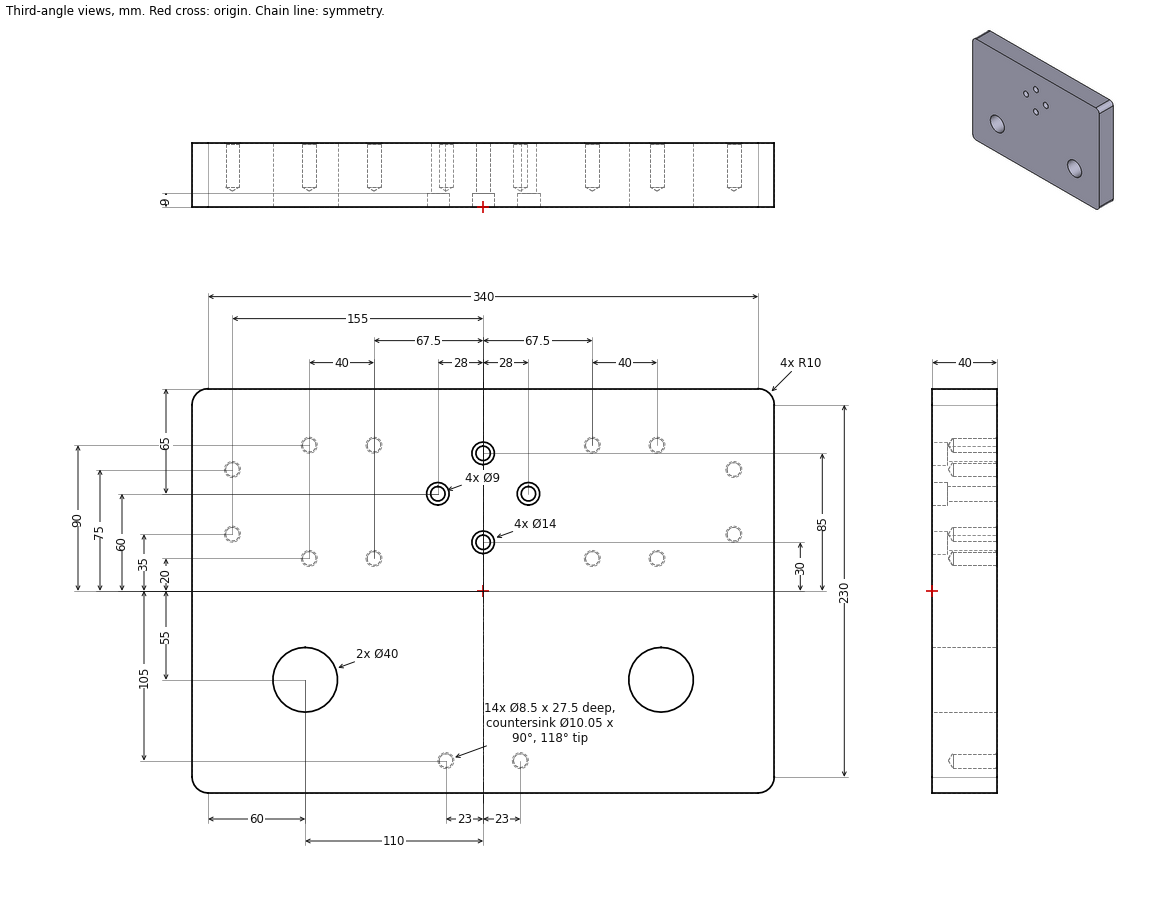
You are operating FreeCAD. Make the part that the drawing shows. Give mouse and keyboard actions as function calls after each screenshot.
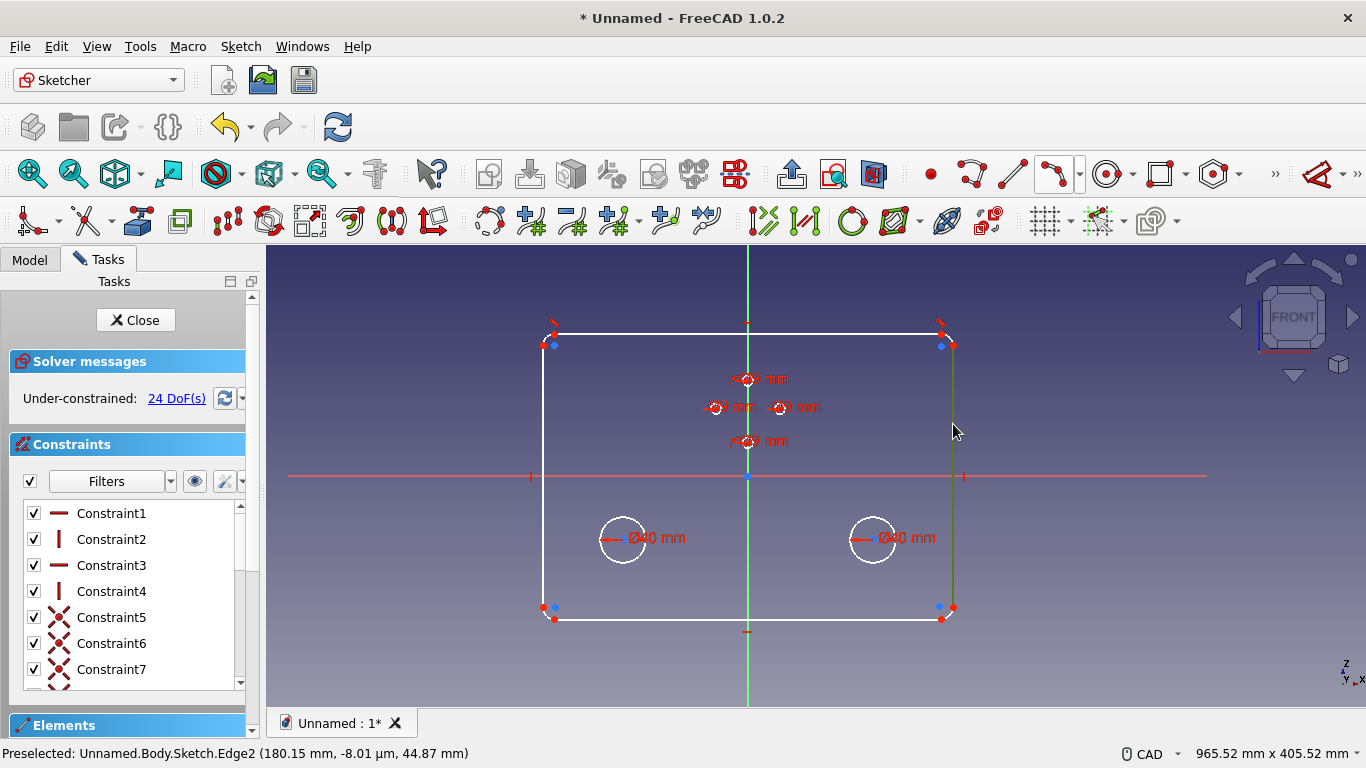
scroll(950, 337, up, 3)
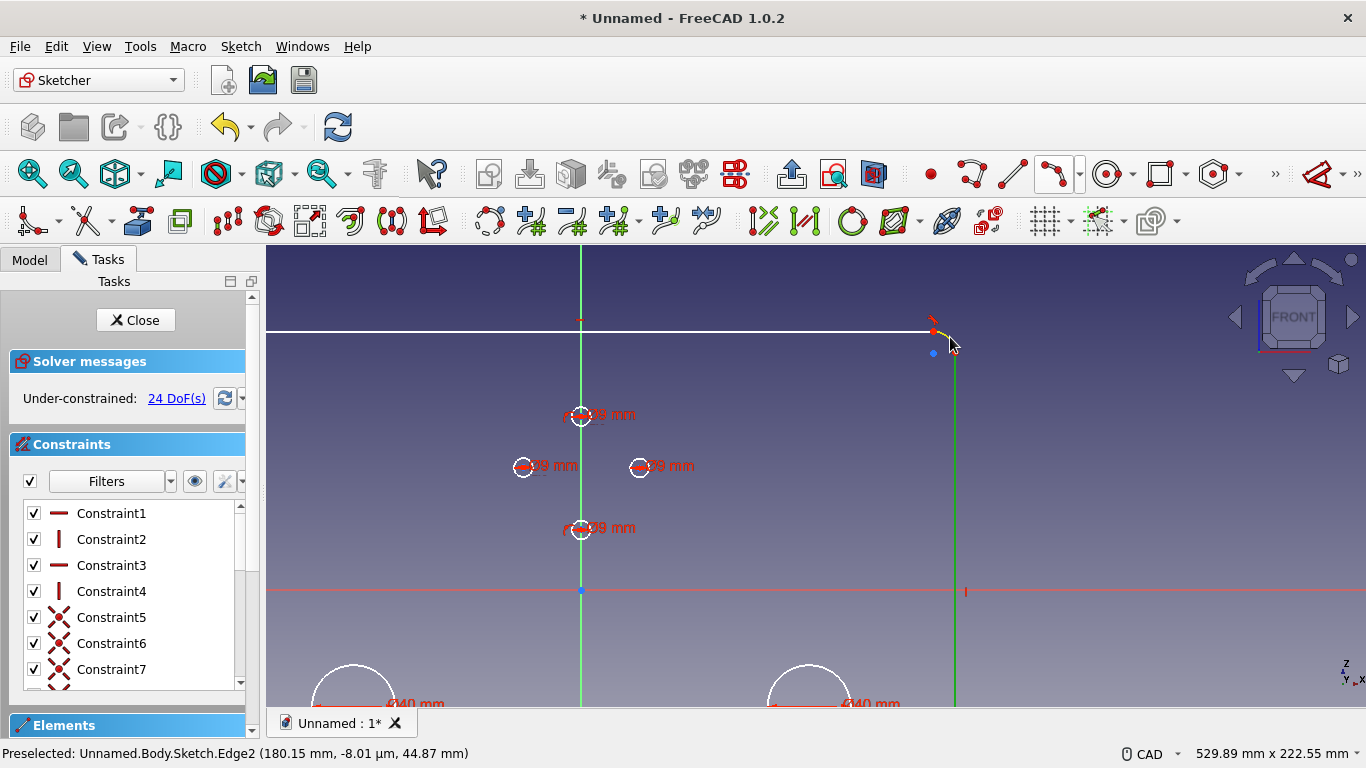
click(949, 338)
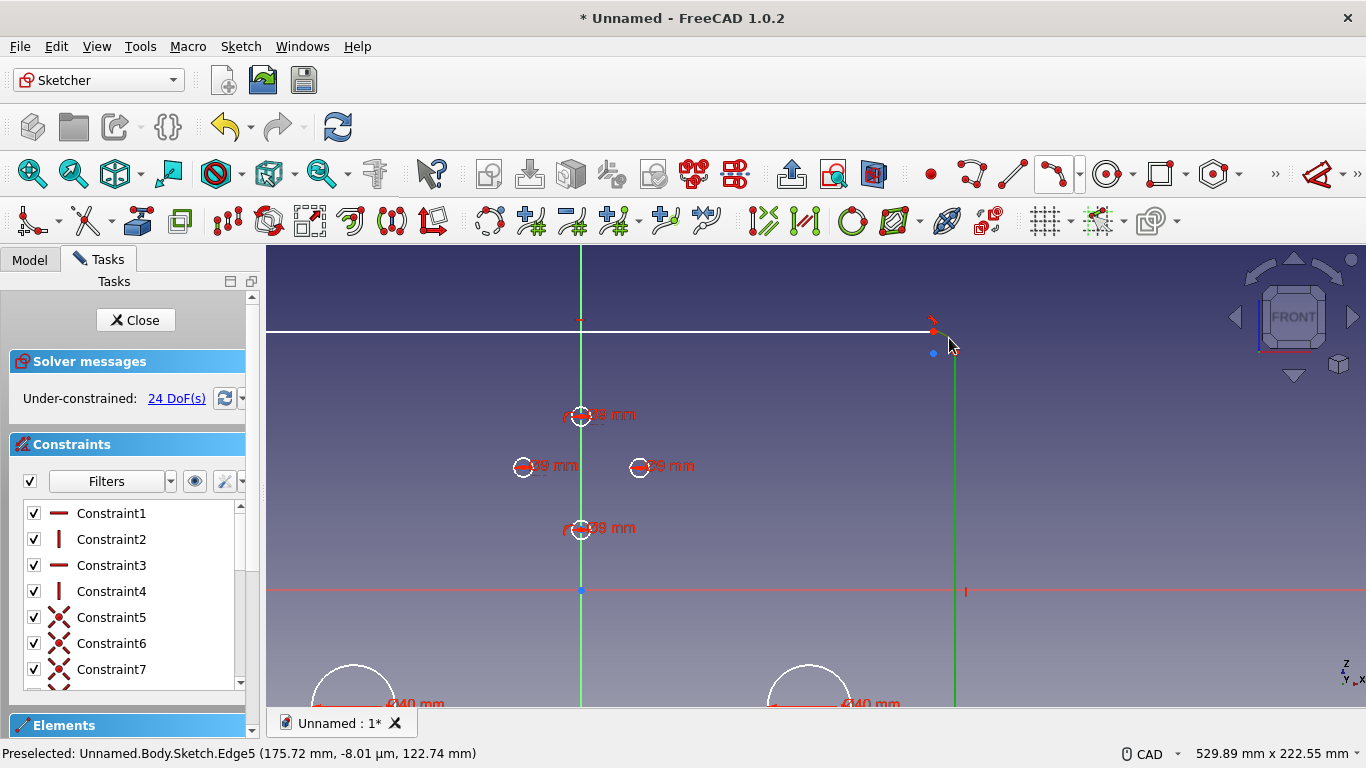
key(t)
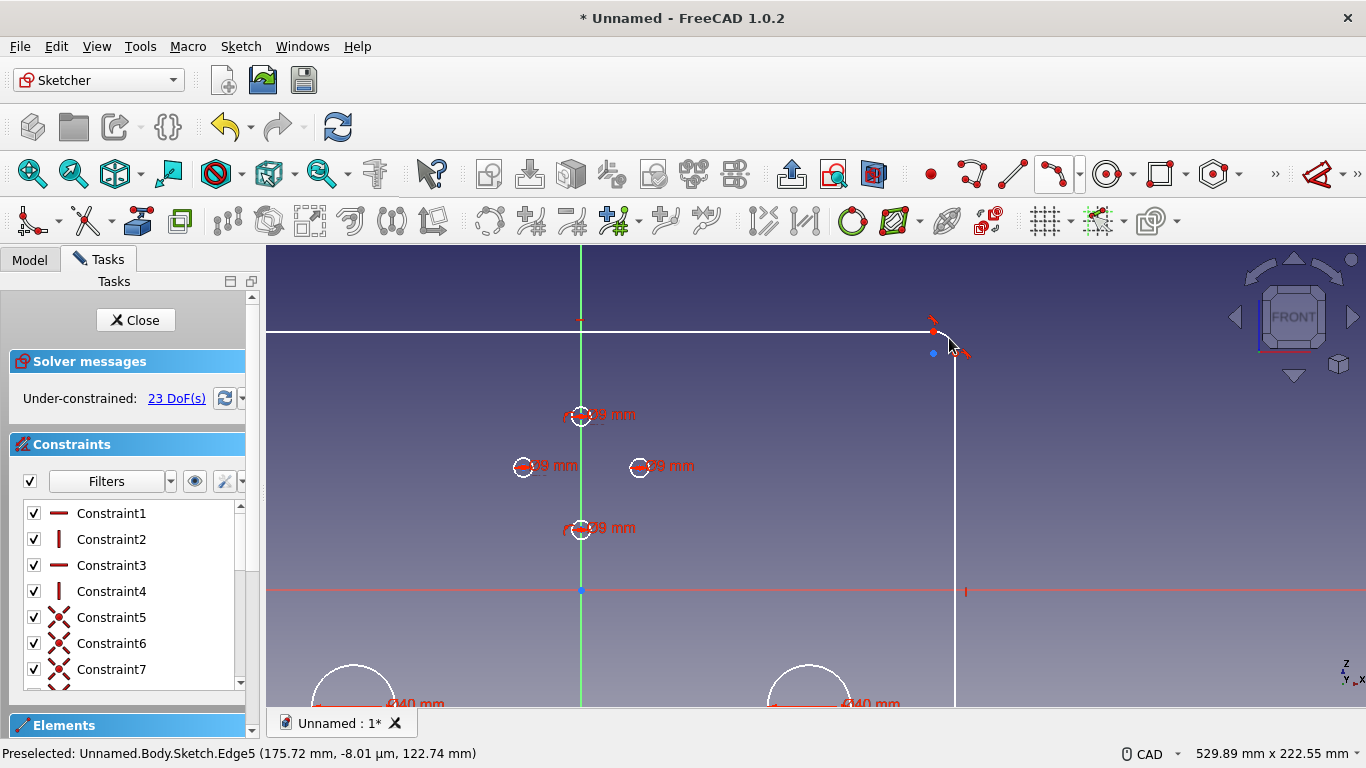
click(955, 496)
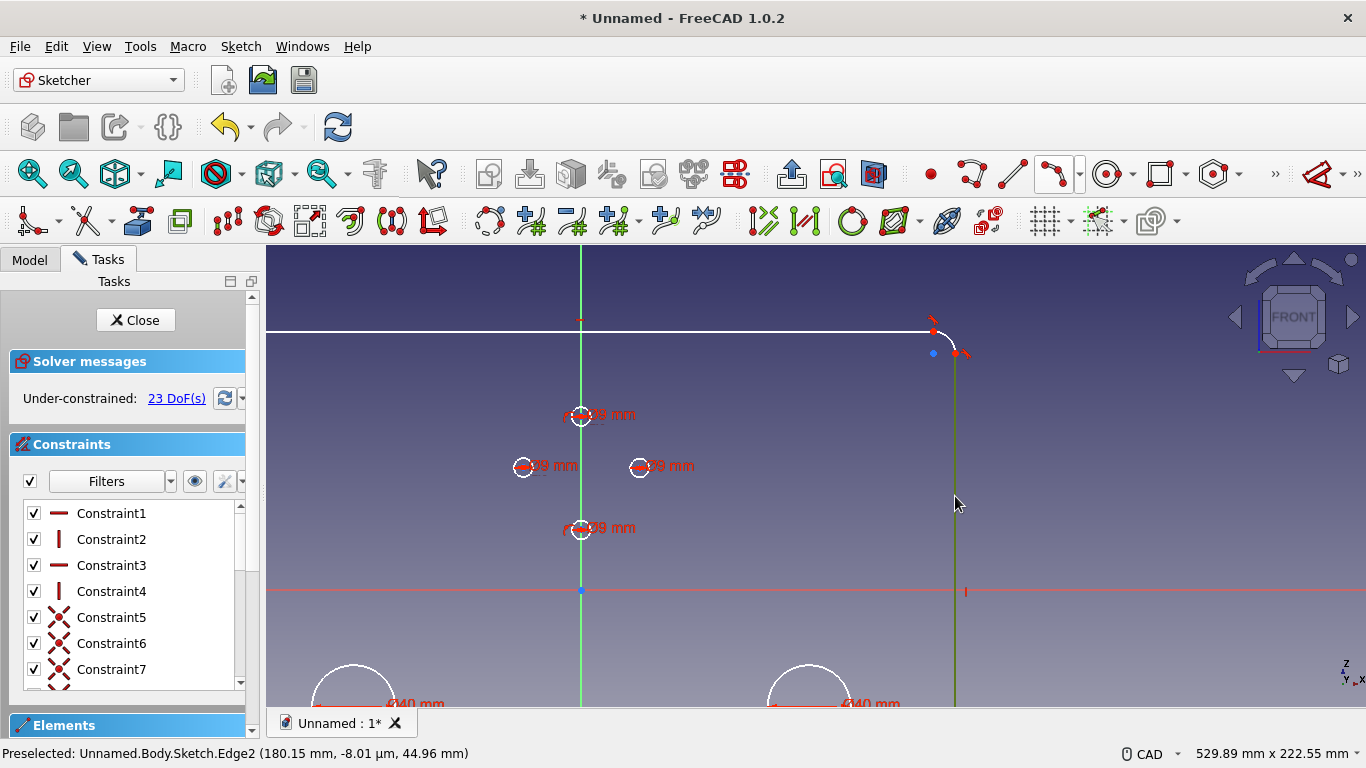
scroll(950, 337, down, 3)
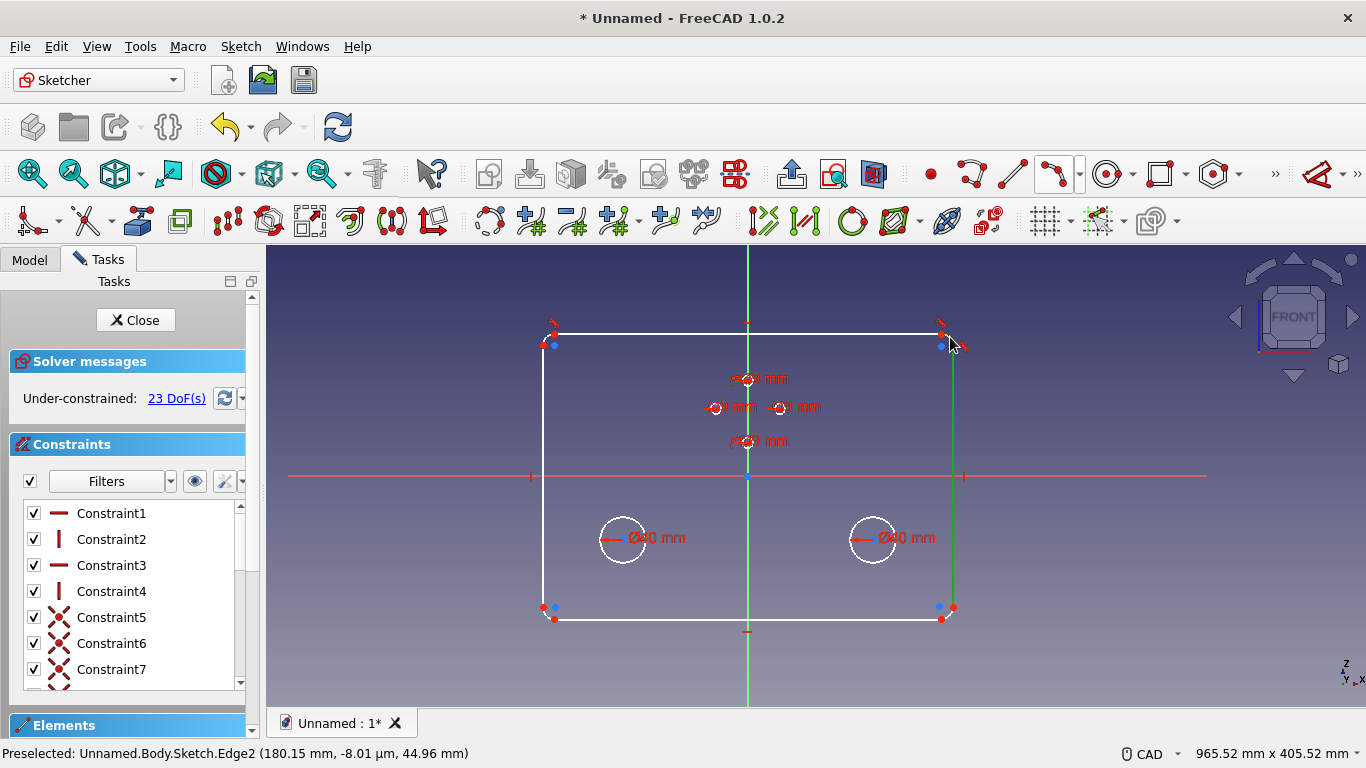
scroll(946, 618, up, 5)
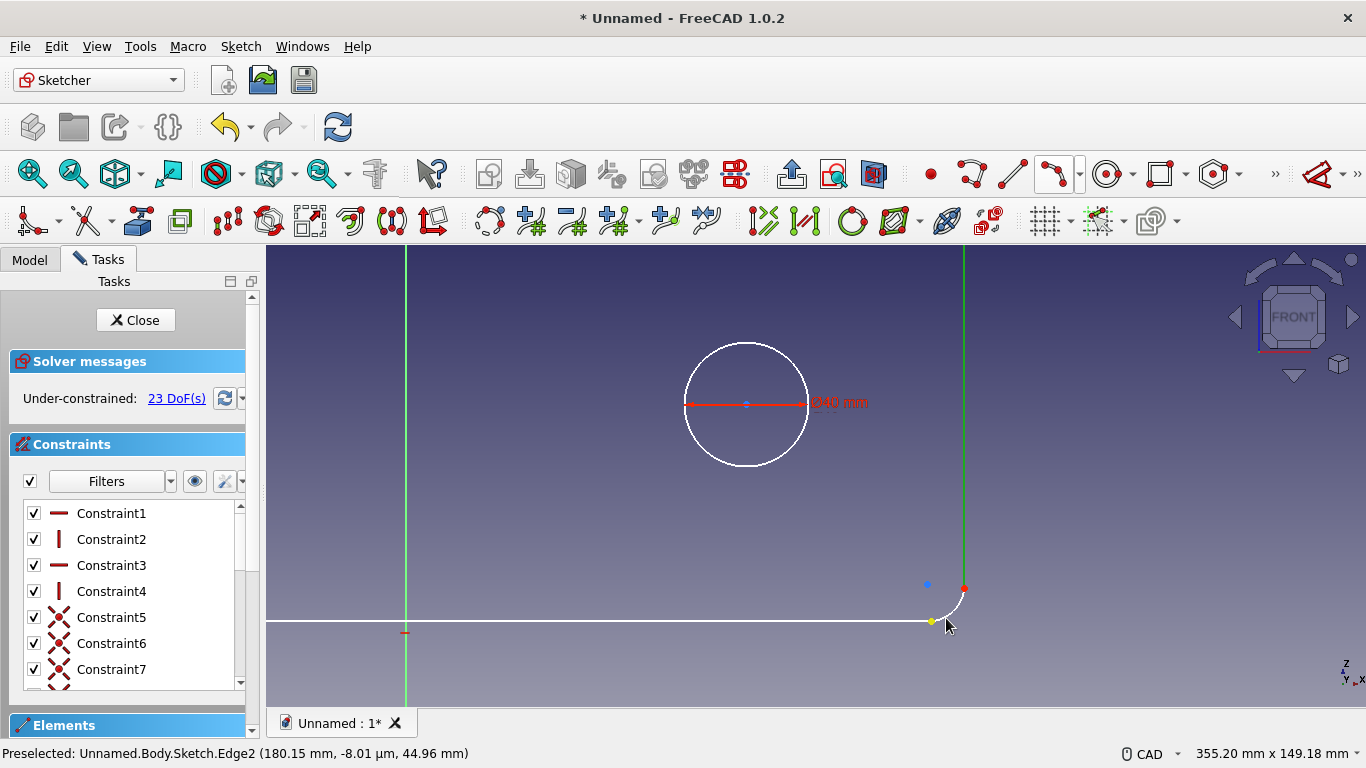
click(946, 617)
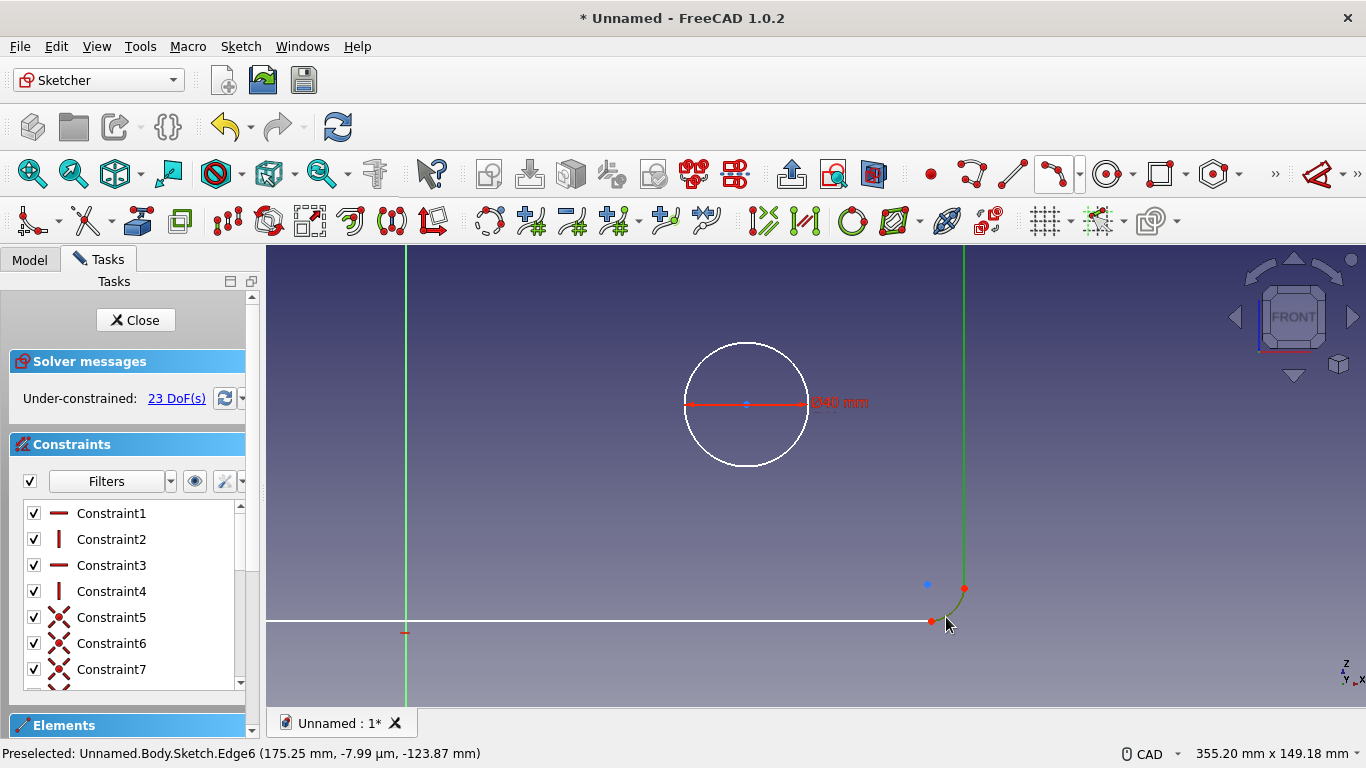
key(t)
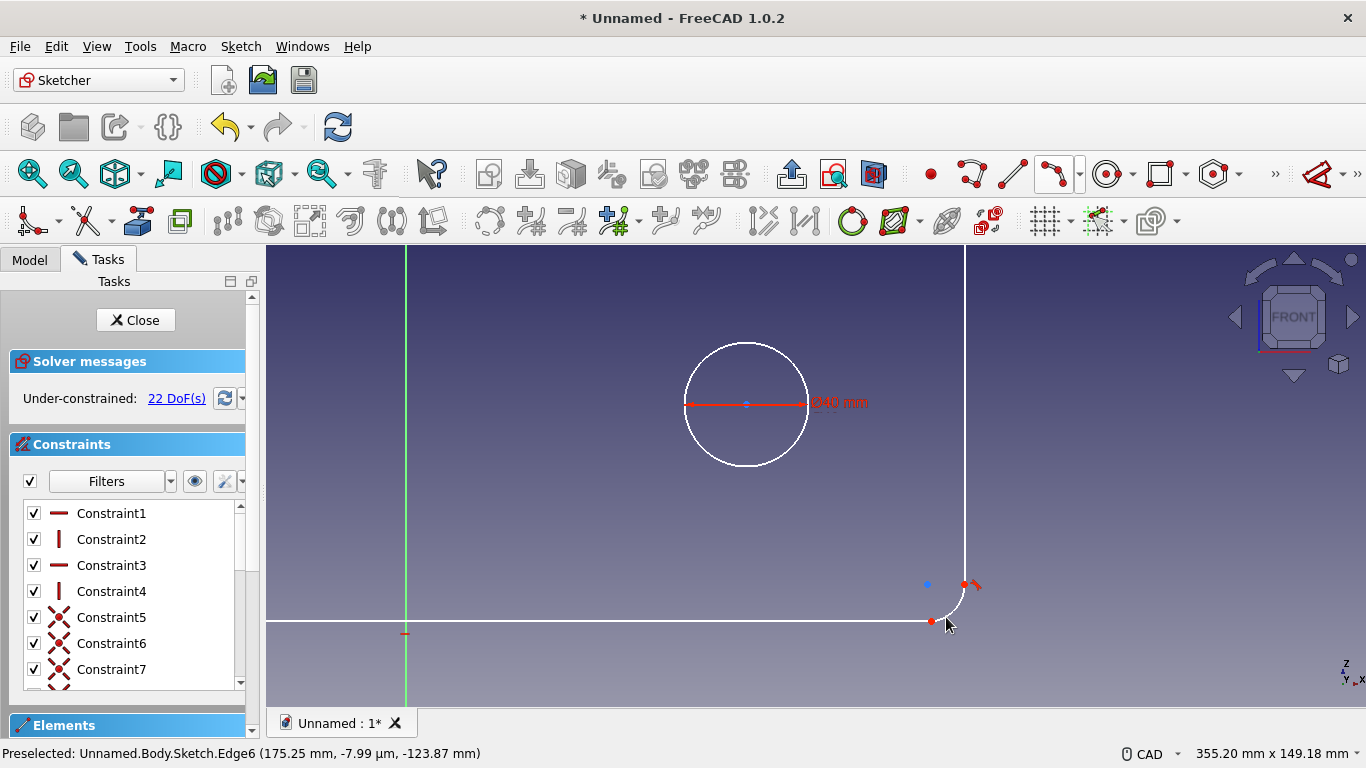
click(616, 621)